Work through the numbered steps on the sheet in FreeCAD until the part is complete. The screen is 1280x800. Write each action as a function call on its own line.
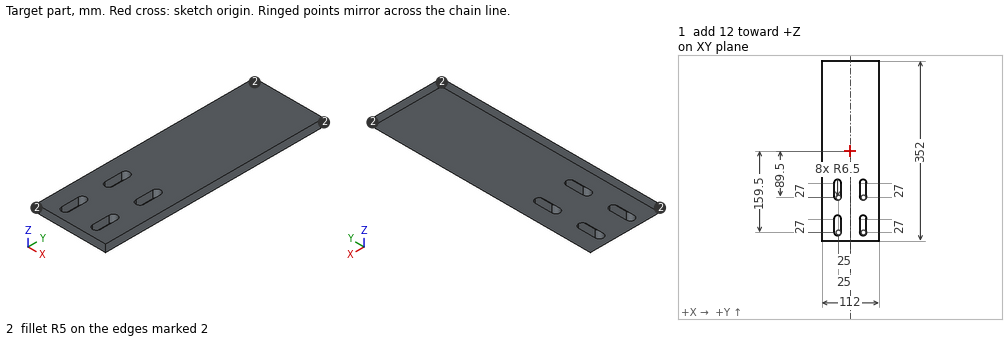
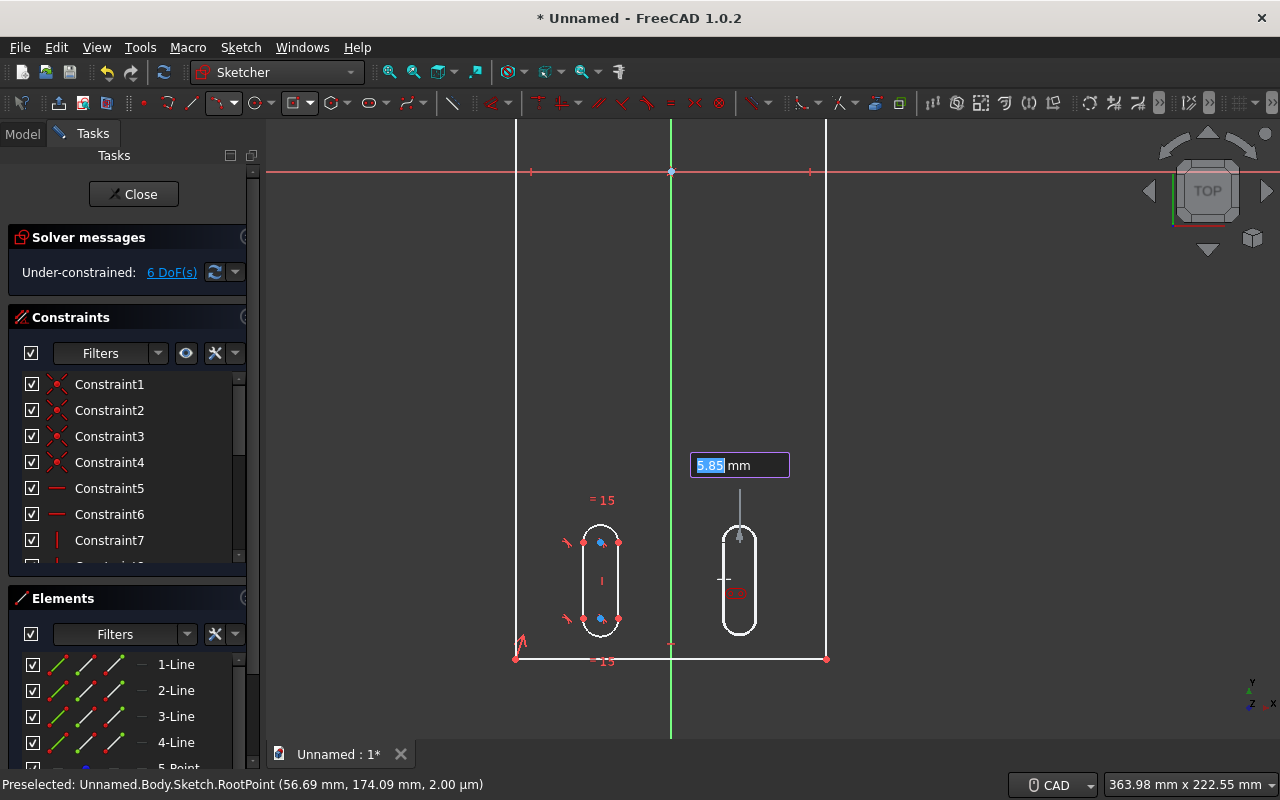
click(723, 578)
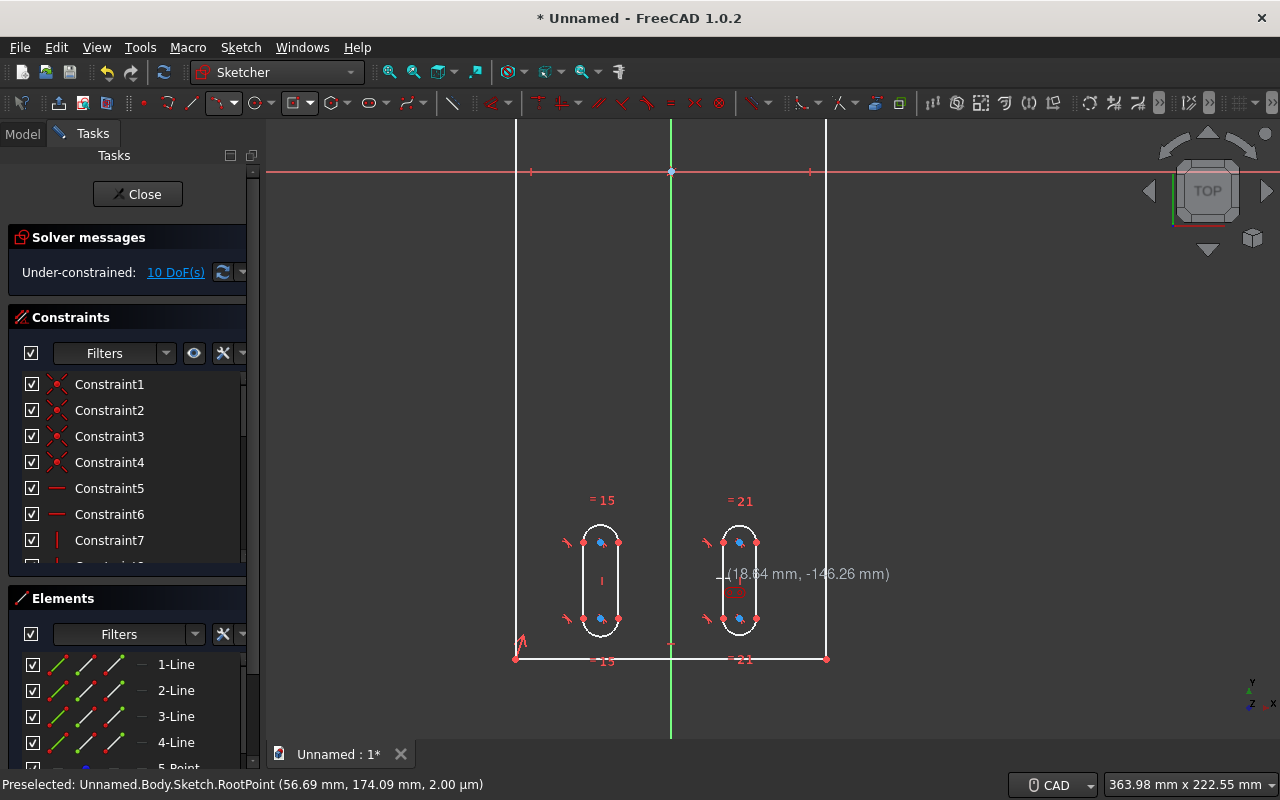
scroll(601, 421, up, 2)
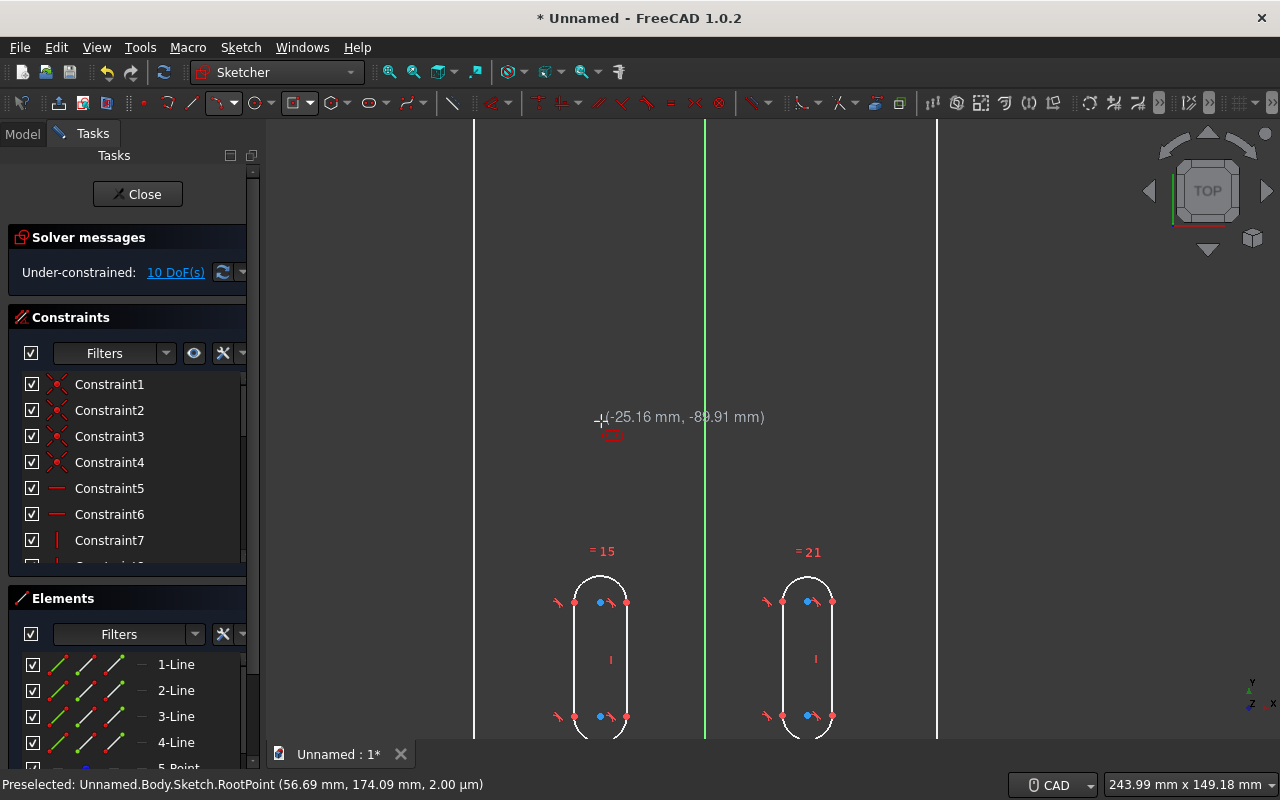
scroll(704, 554, down, 7)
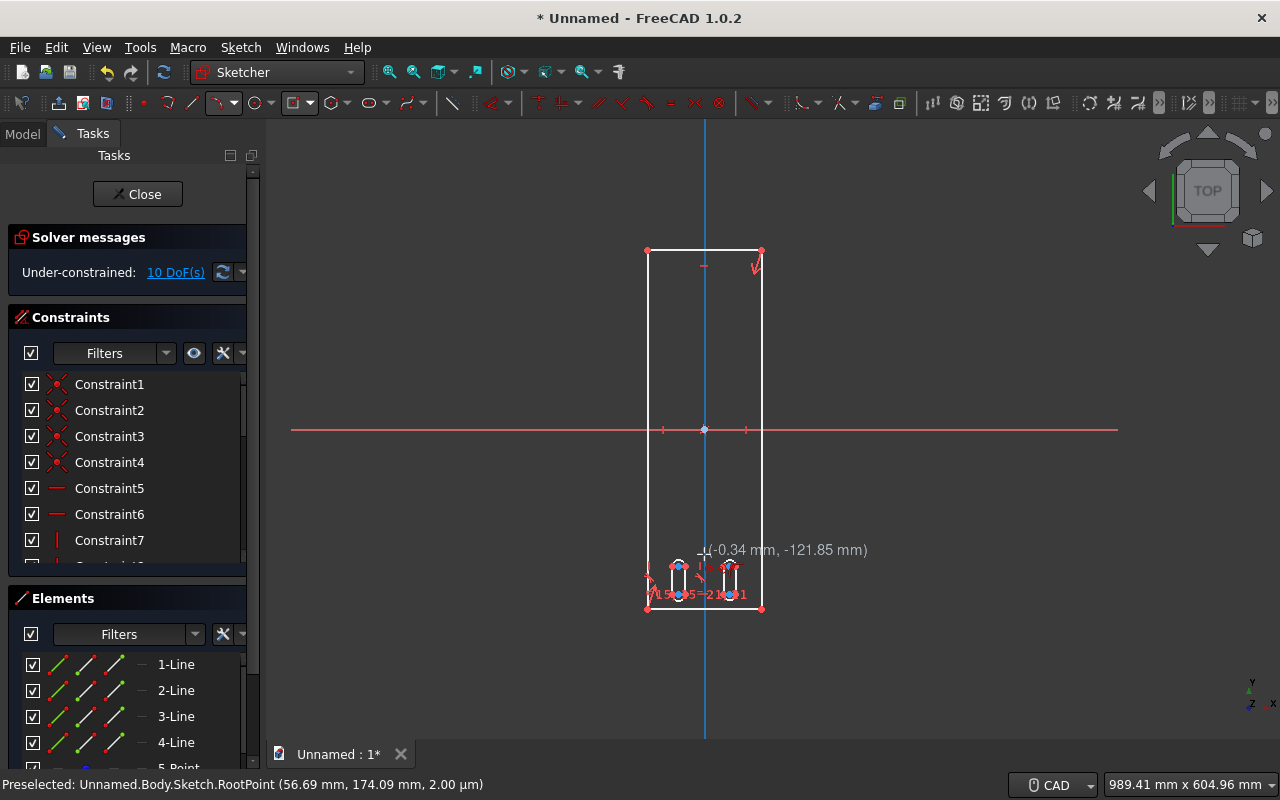
click(679, 522)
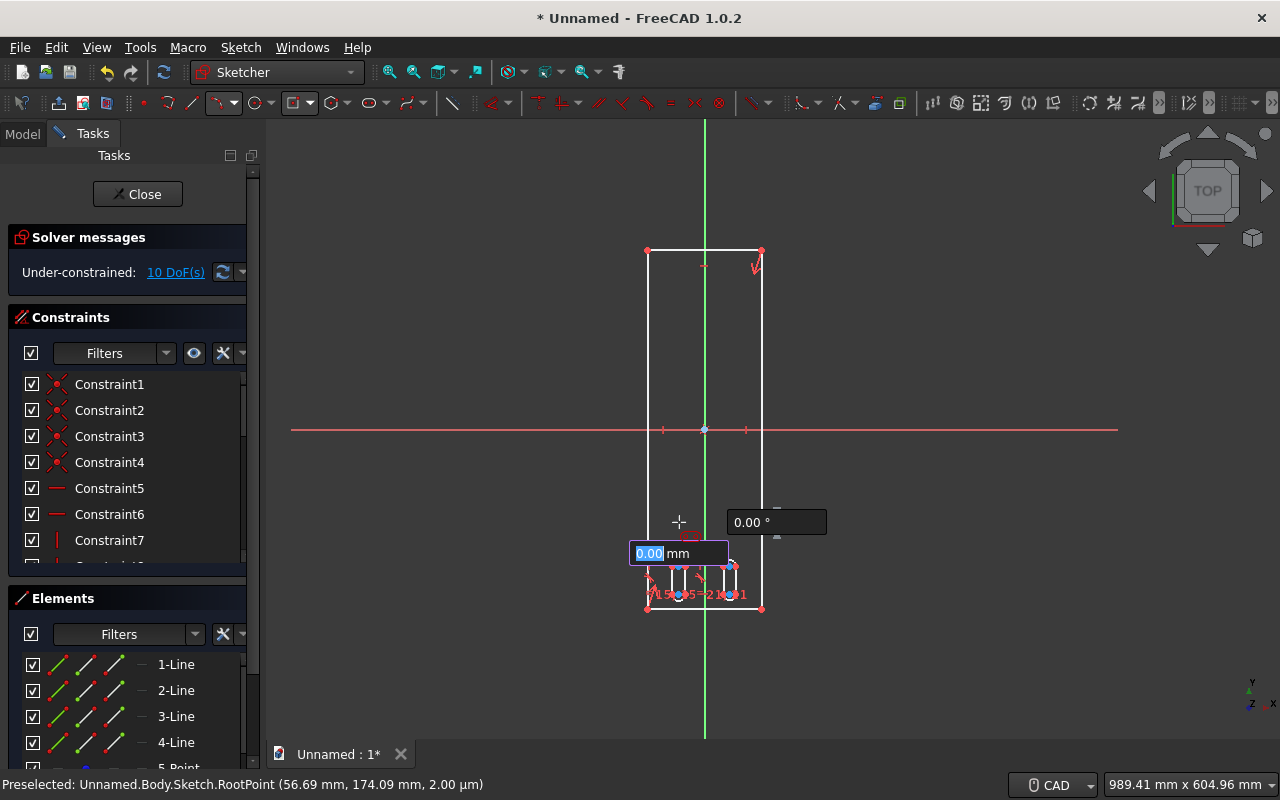
click(679, 494)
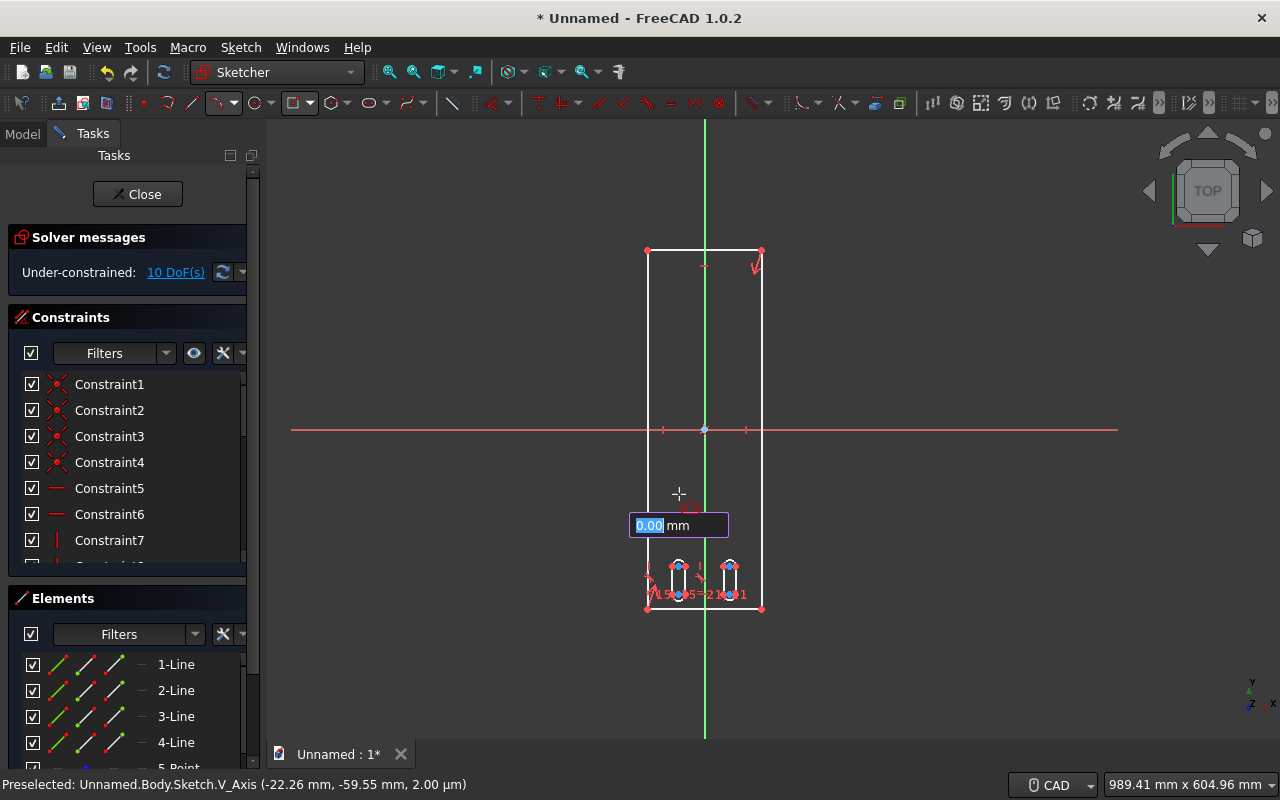
scroll(686, 508, up, 5)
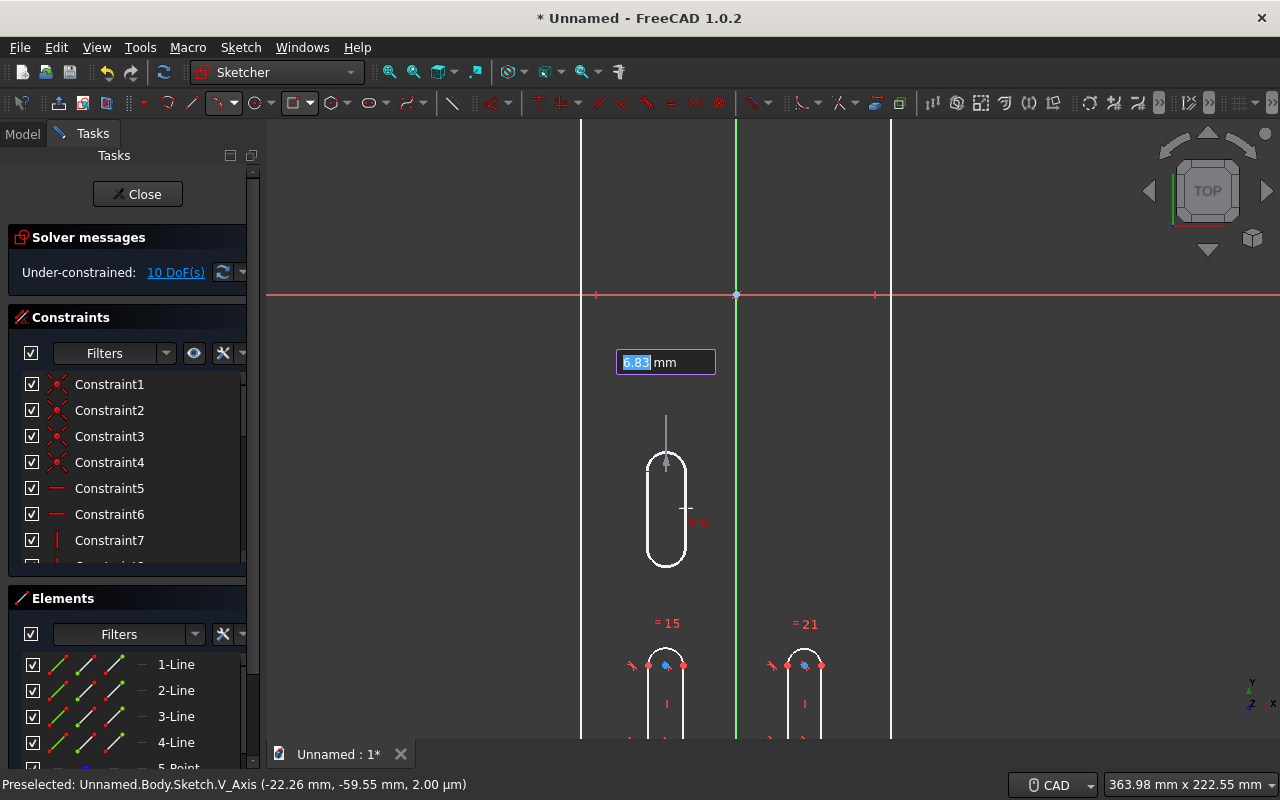
click(684, 506)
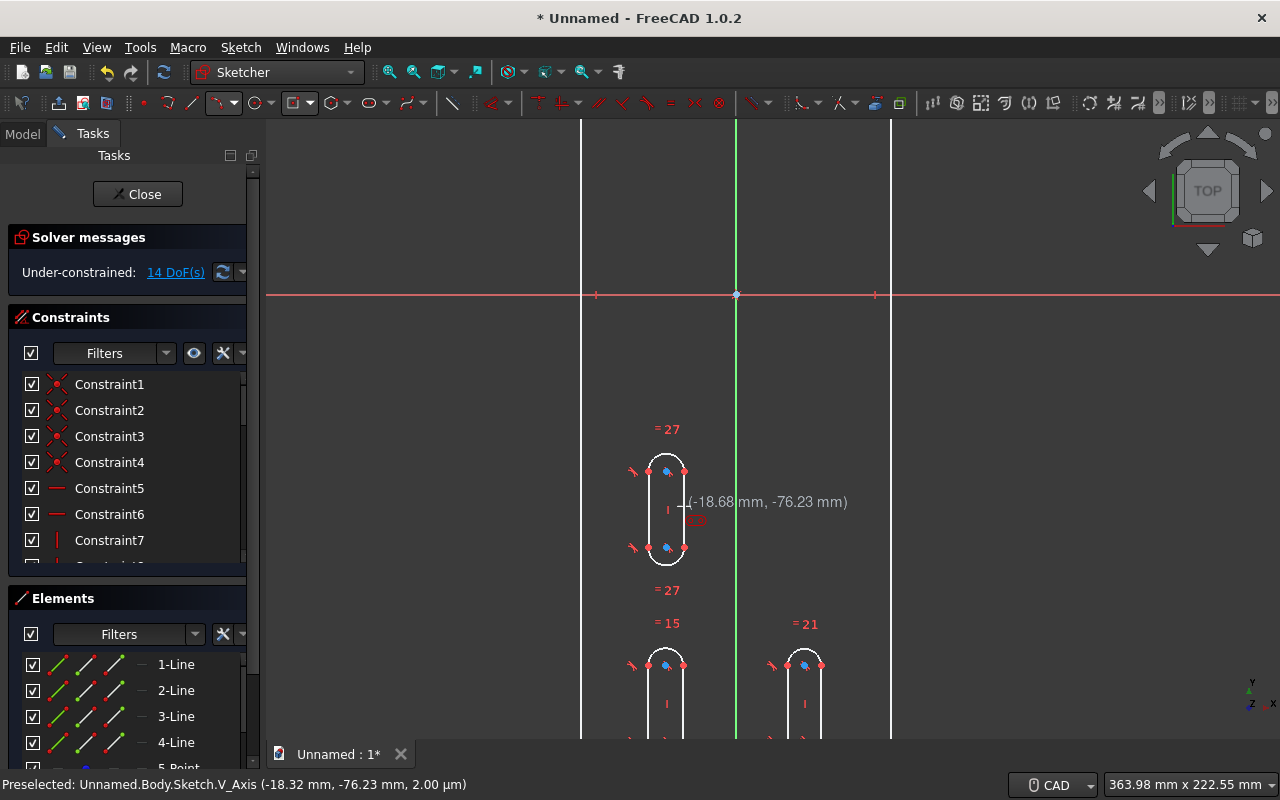
scroll(806, 544, up, 2)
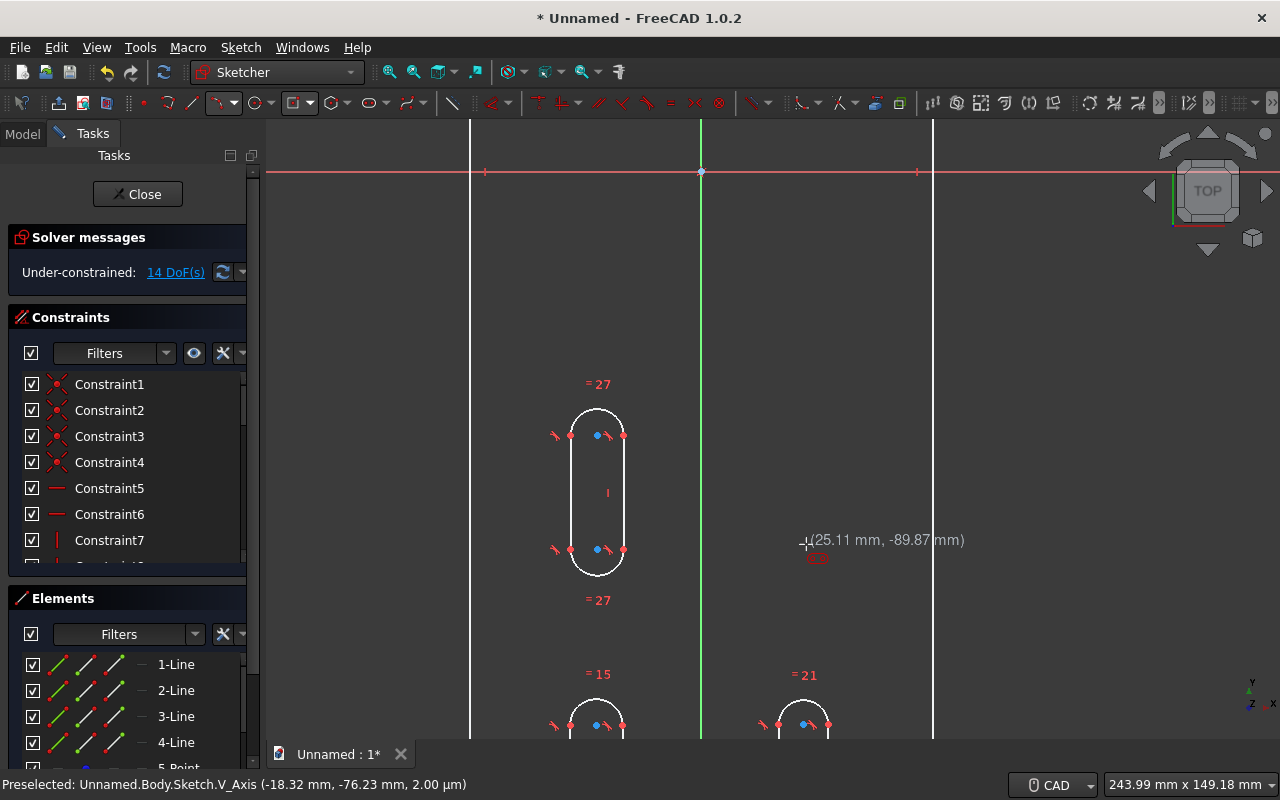
scroll(706, 513, down, 7)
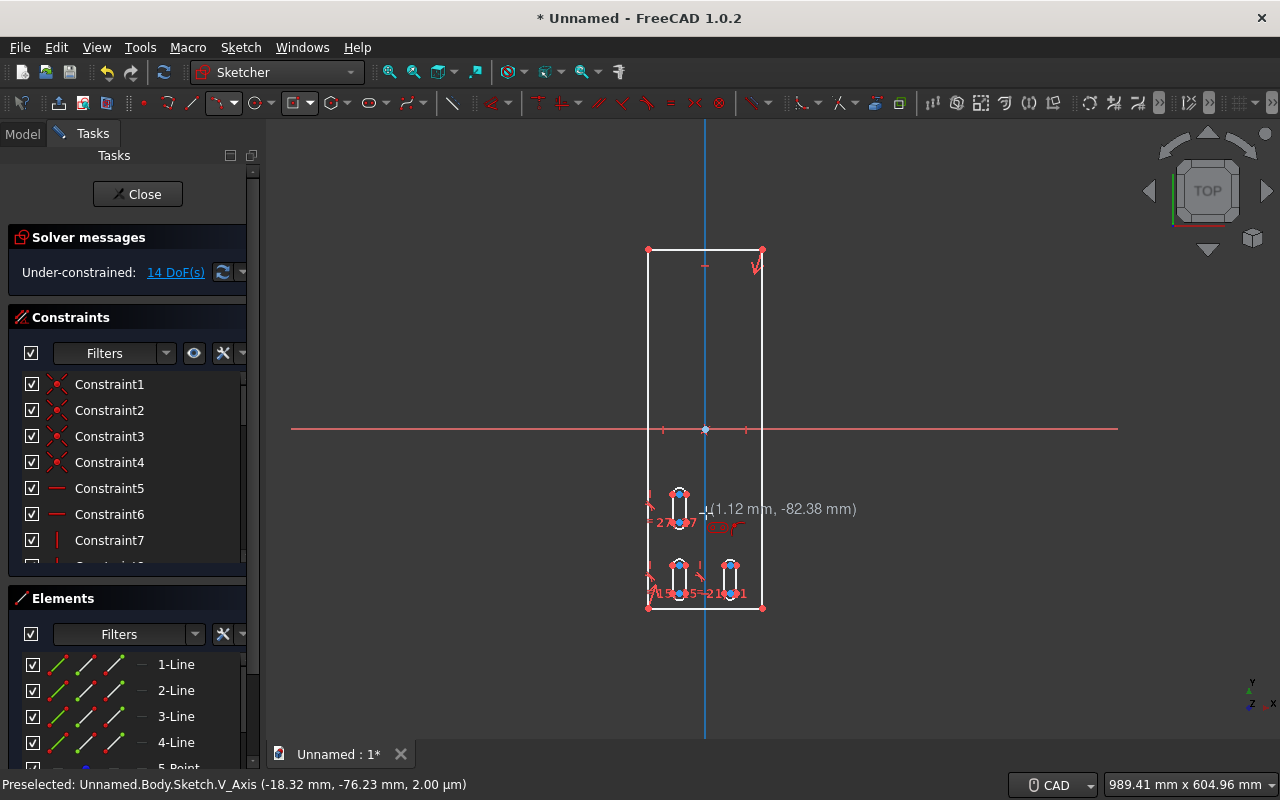
click(731, 521)